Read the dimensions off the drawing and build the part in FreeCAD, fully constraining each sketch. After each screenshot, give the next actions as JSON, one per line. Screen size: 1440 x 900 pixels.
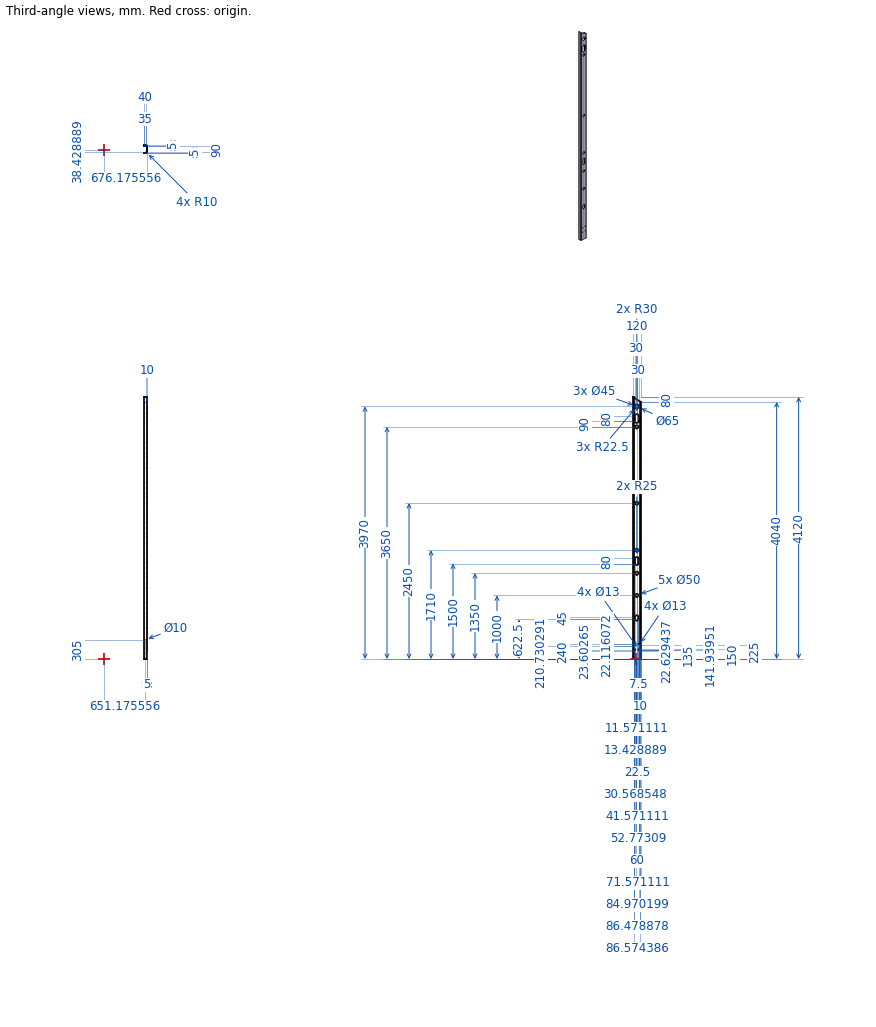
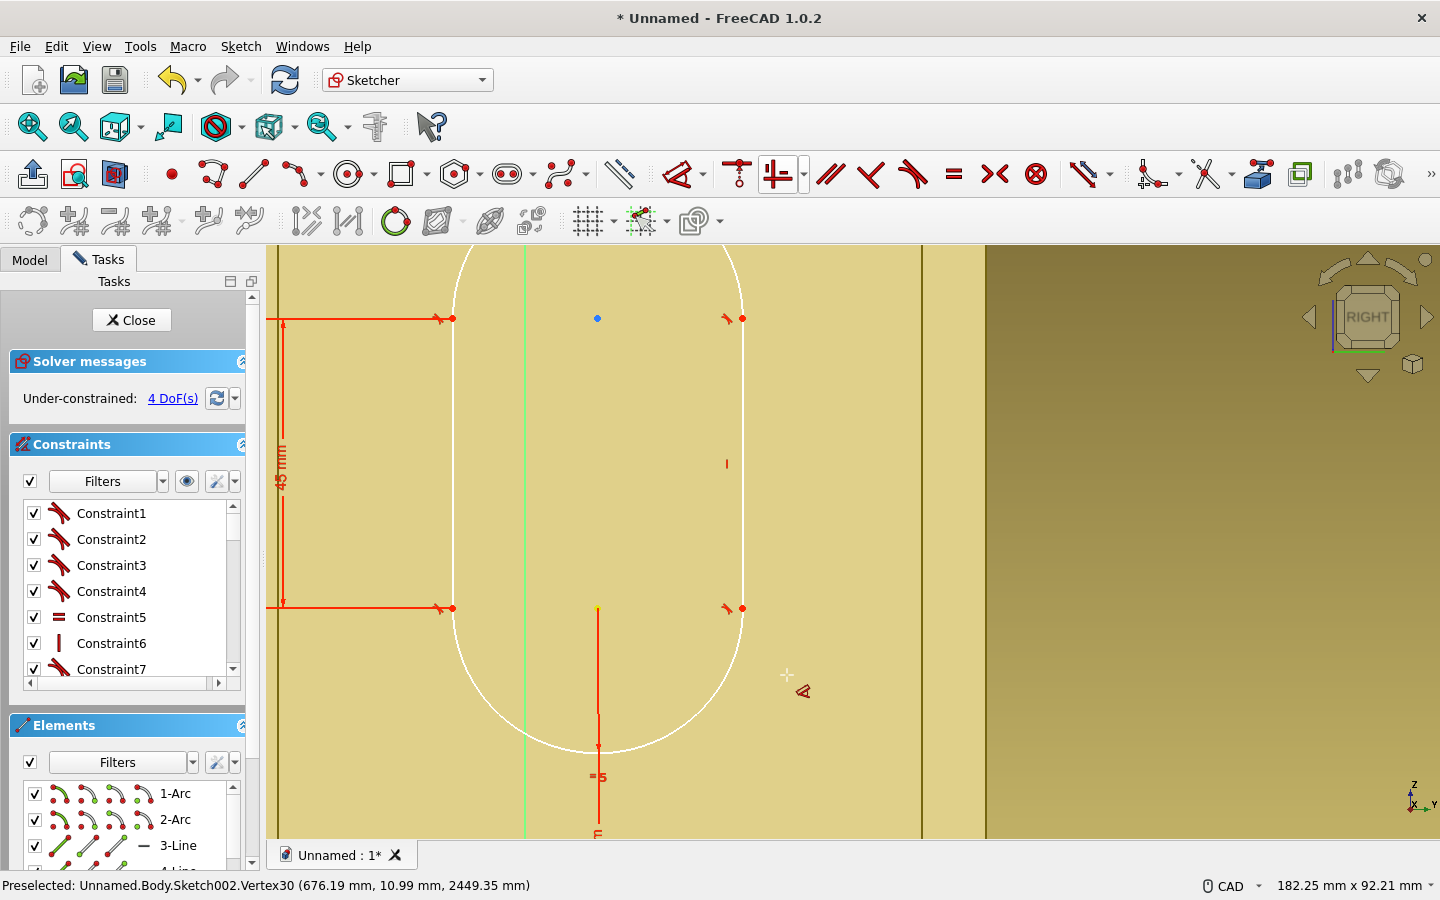
{"action": "left_click", "coordinate": [743, 608]}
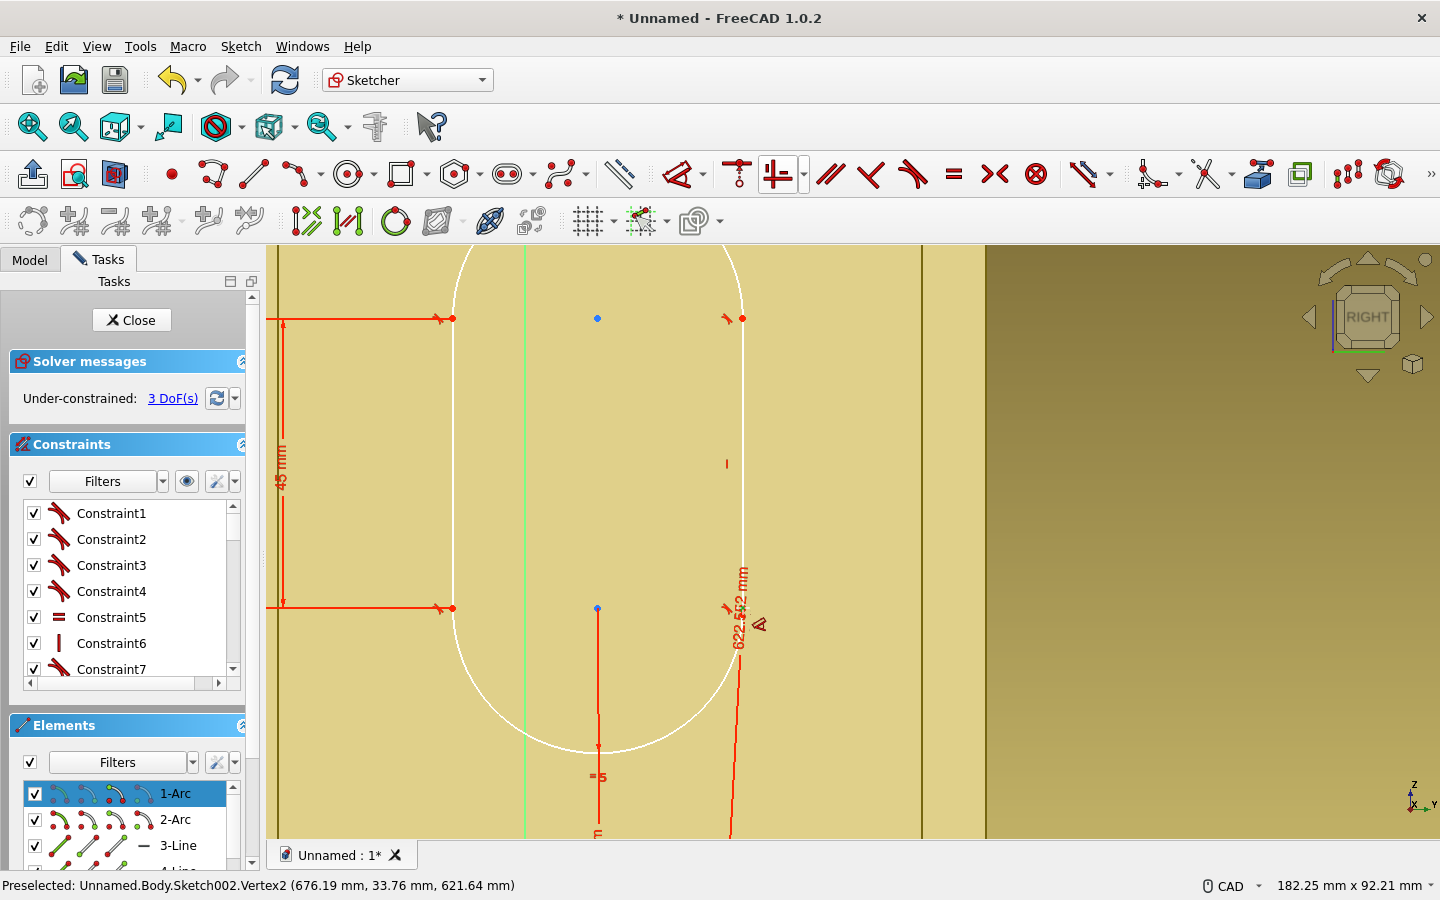
{"action": "scroll", "coordinate": [784, 542], "scroll_direction": "down", "scroll_amount": 15}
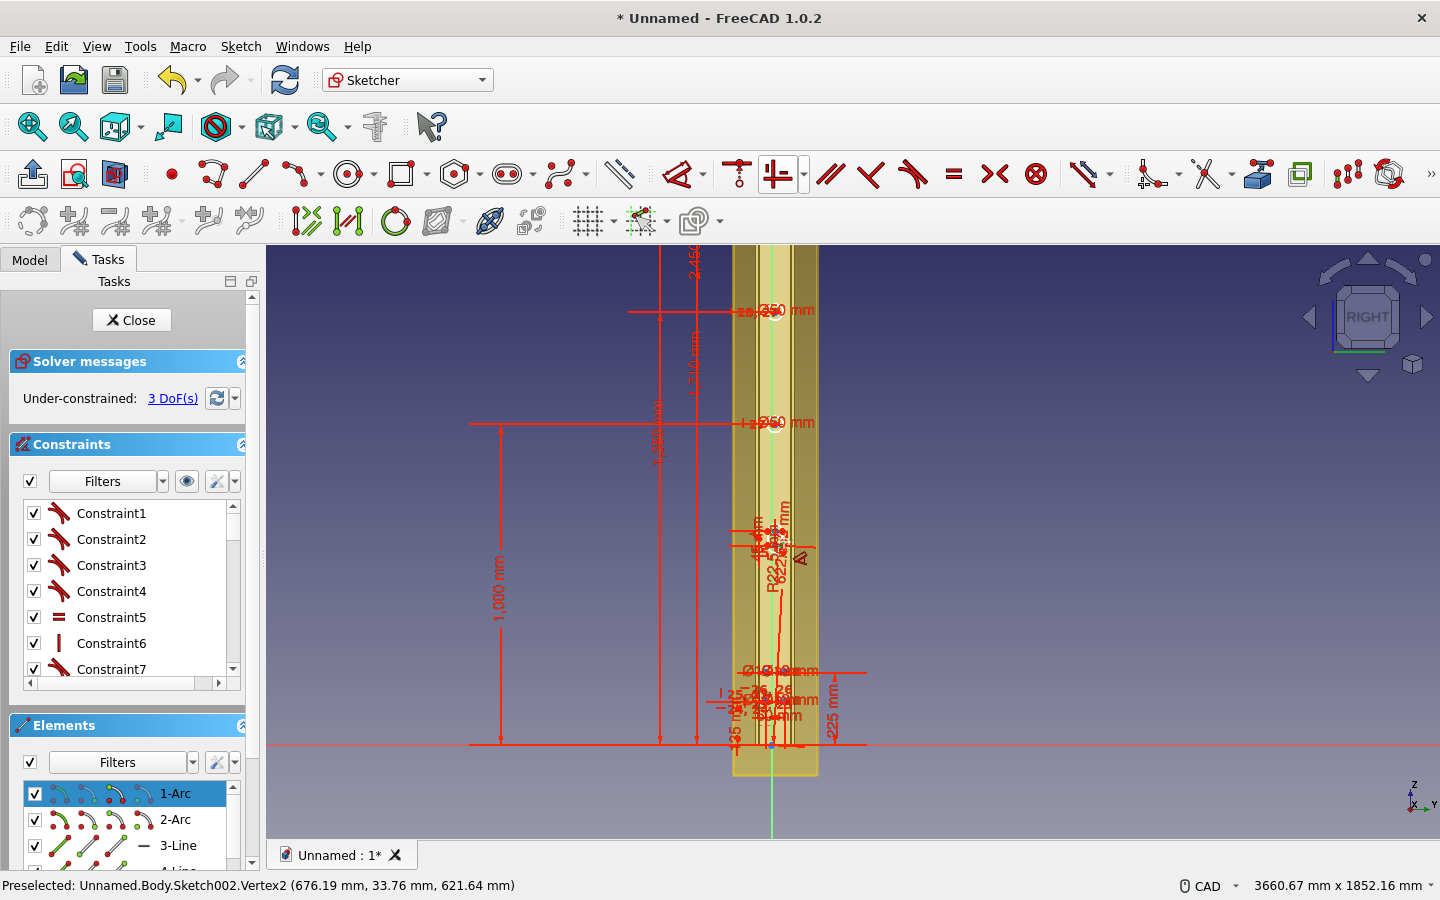
{"action": "scroll", "coordinate": [788, 730], "scroll_direction": "down", "scroll_amount": 6}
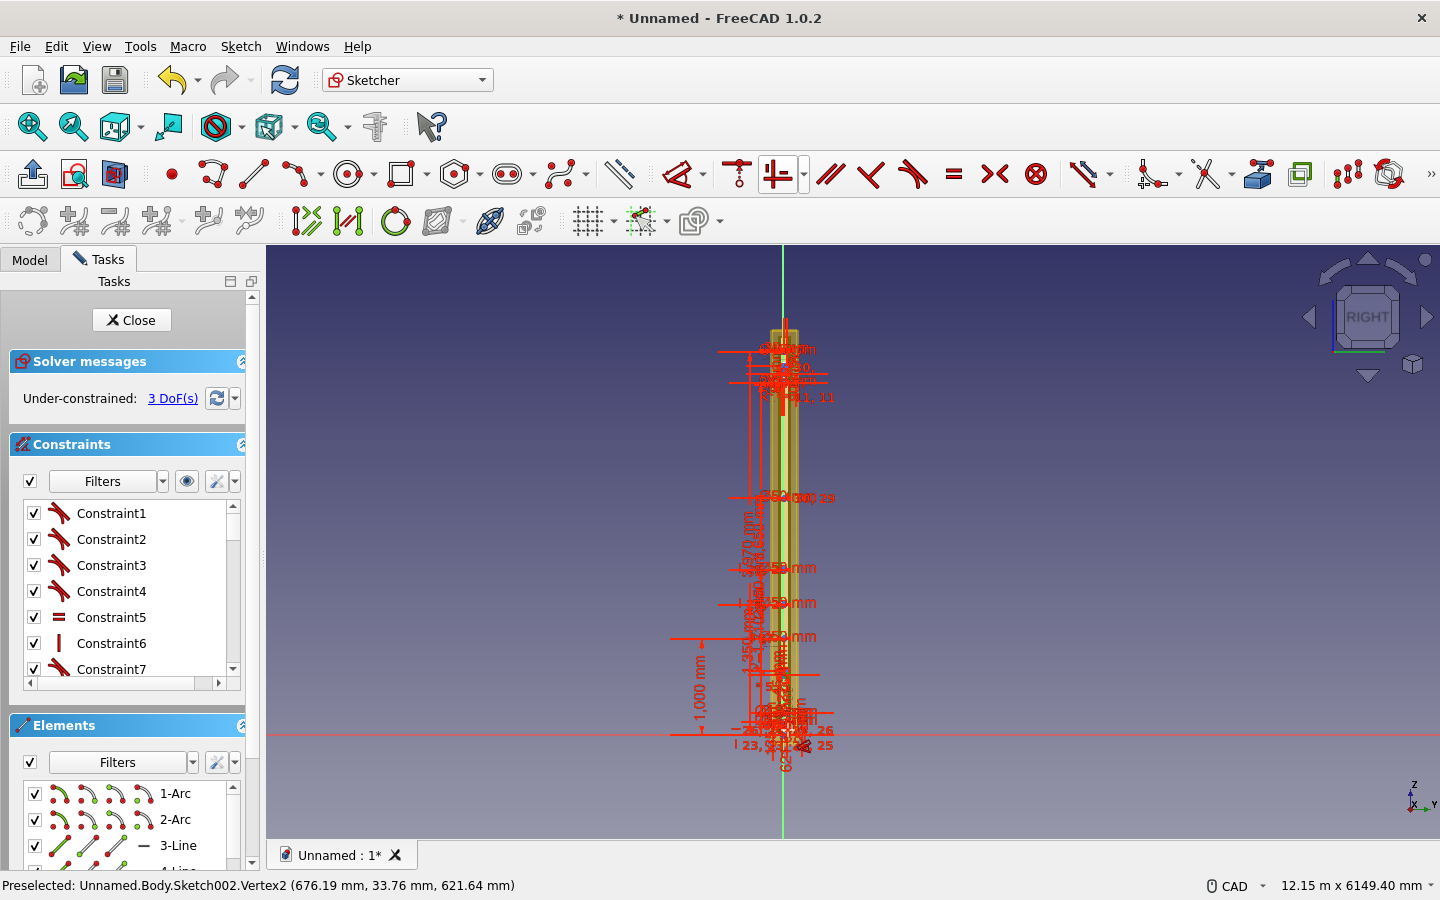
{"action": "scroll", "coordinate": [787, 713], "scroll_direction": "up", "scroll_amount": 21}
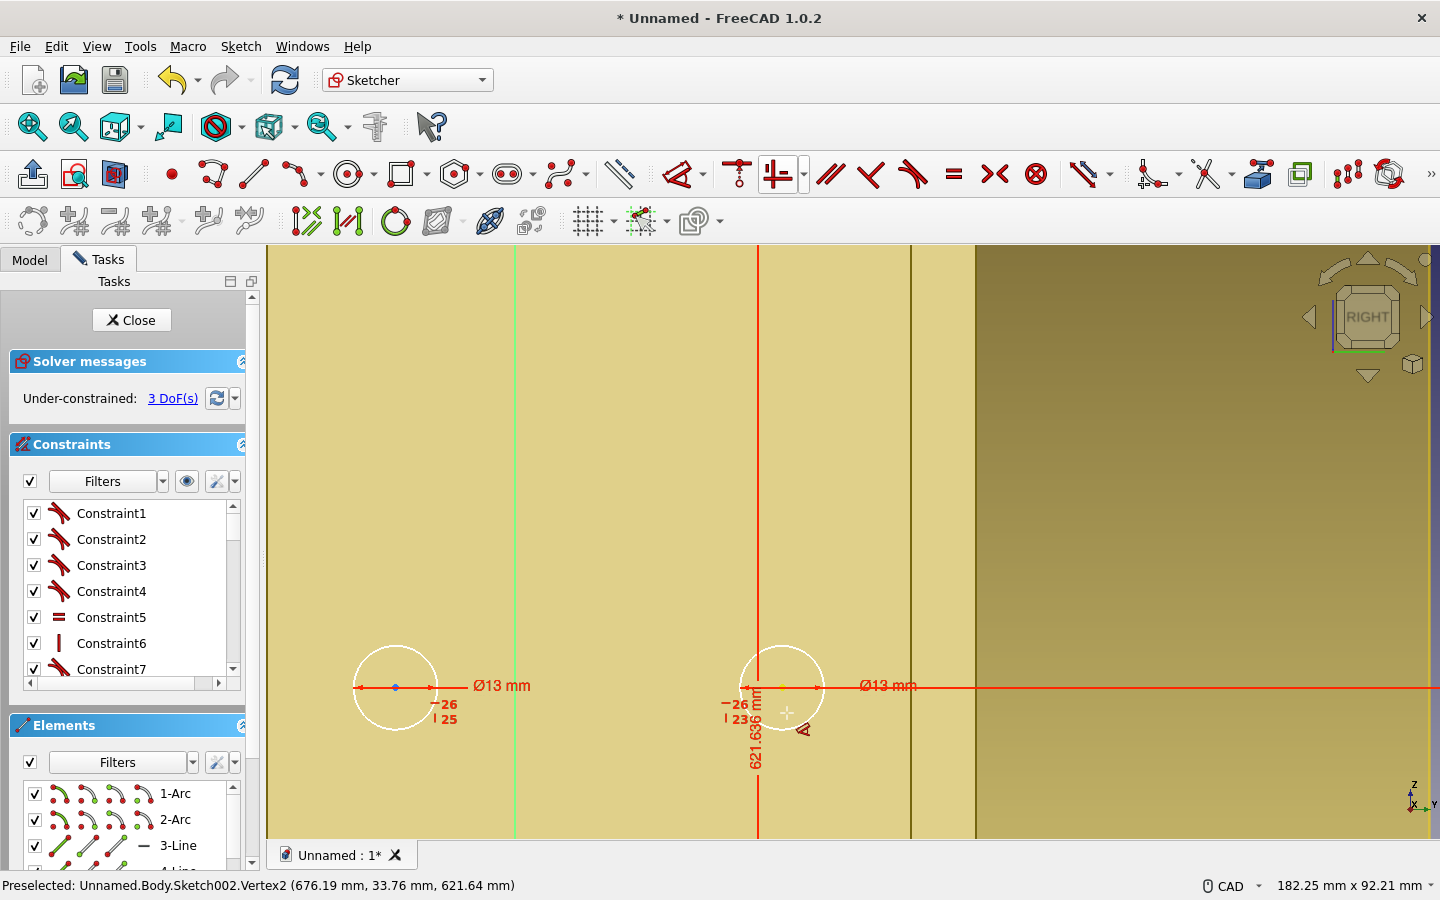
{"action": "left_click", "coordinate": [782, 688]}
{"action": "left_click", "coordinate": [757, 746]}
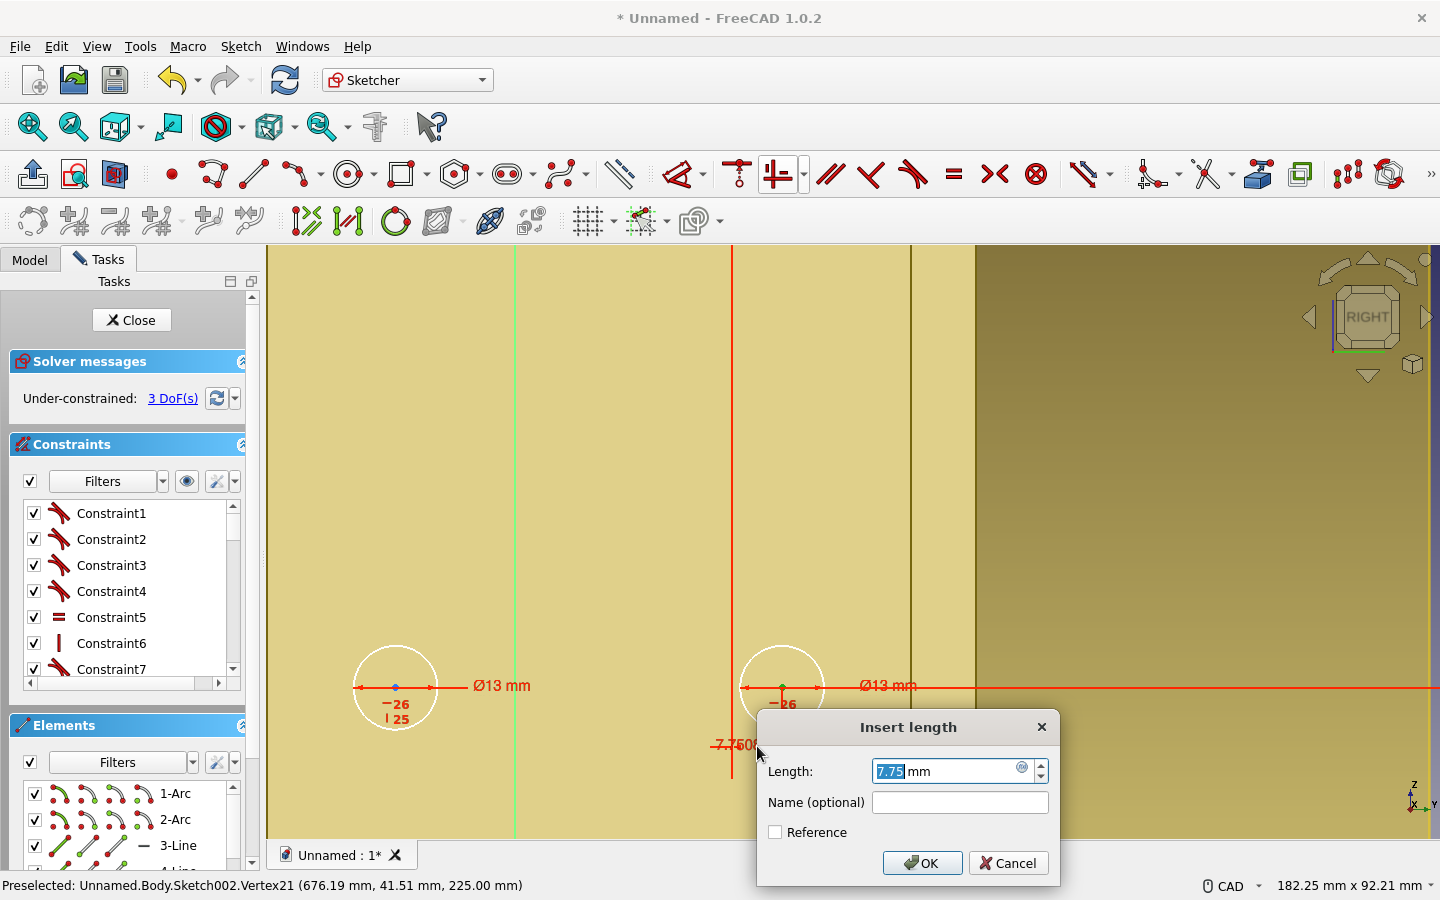
{"action": "type", "text": "7.5"}
{"action": "key", "text": "Return"}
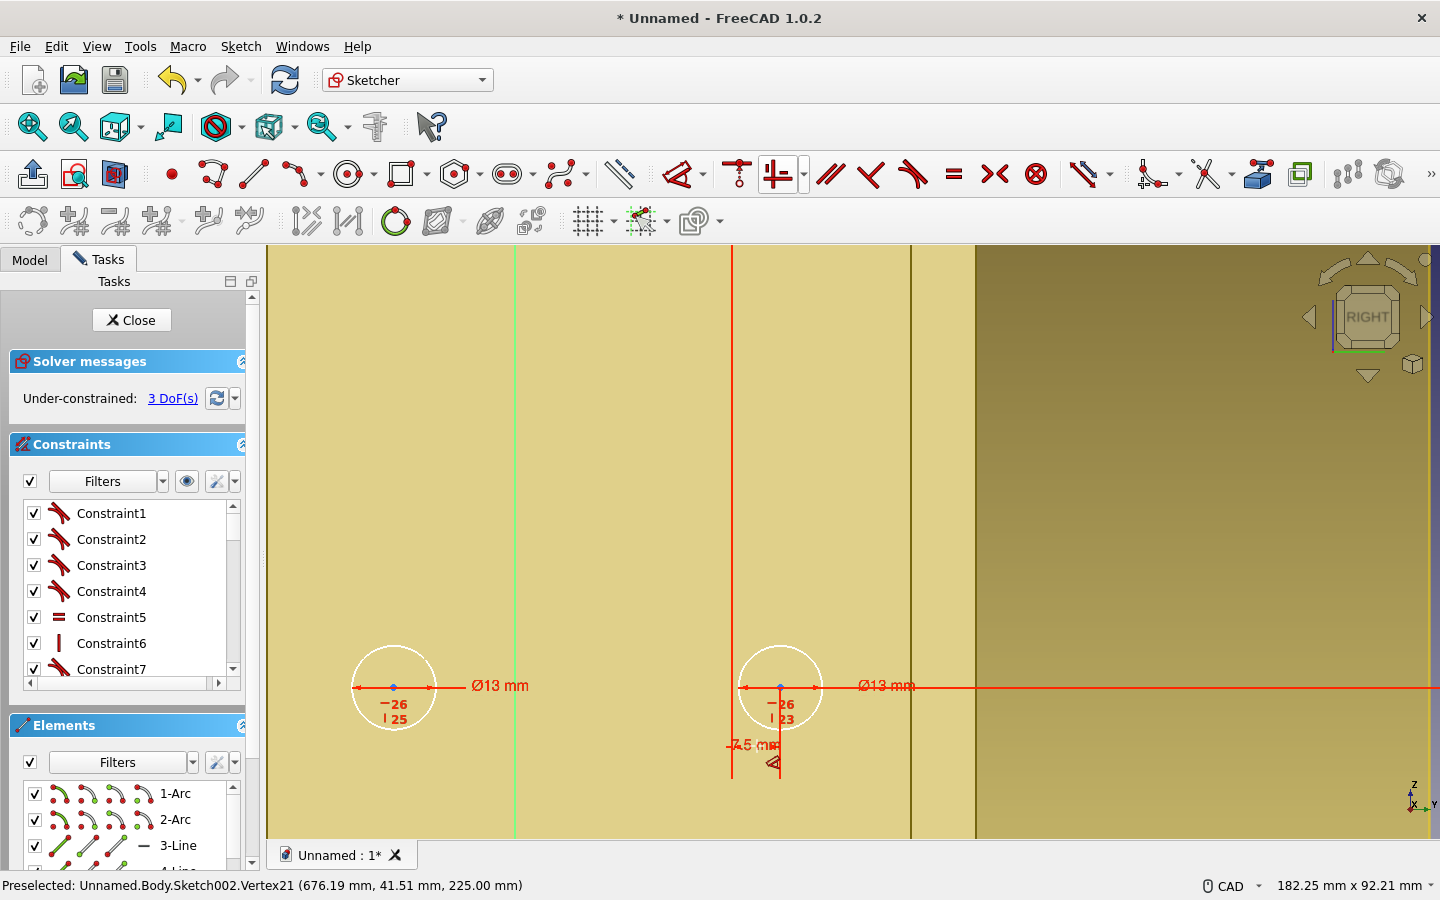
{"action": "scroll", "coordinate": [784, 542], "scroll_direction": "down", "scroll_amount": 15}